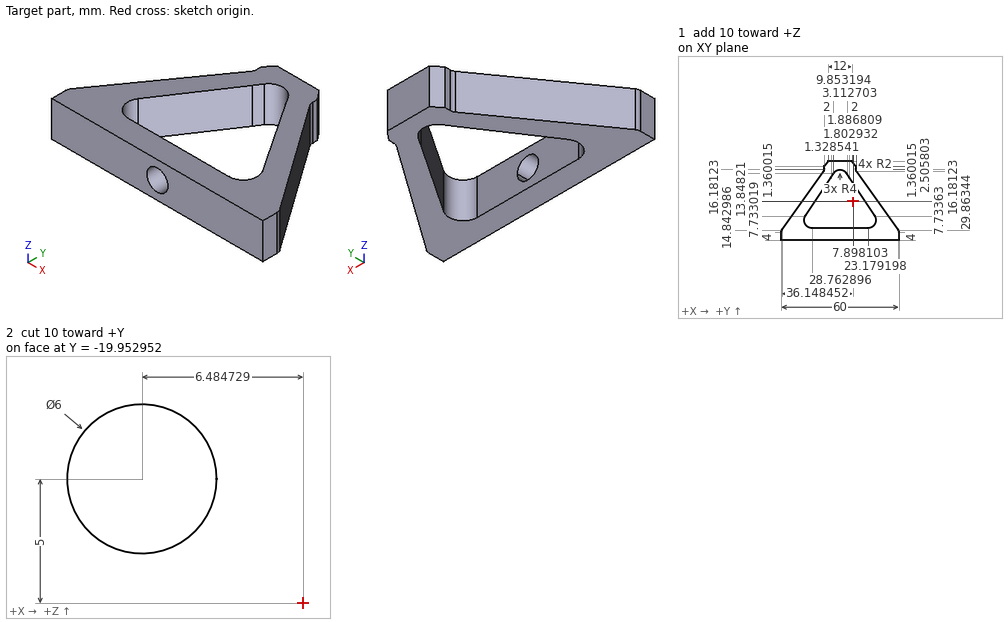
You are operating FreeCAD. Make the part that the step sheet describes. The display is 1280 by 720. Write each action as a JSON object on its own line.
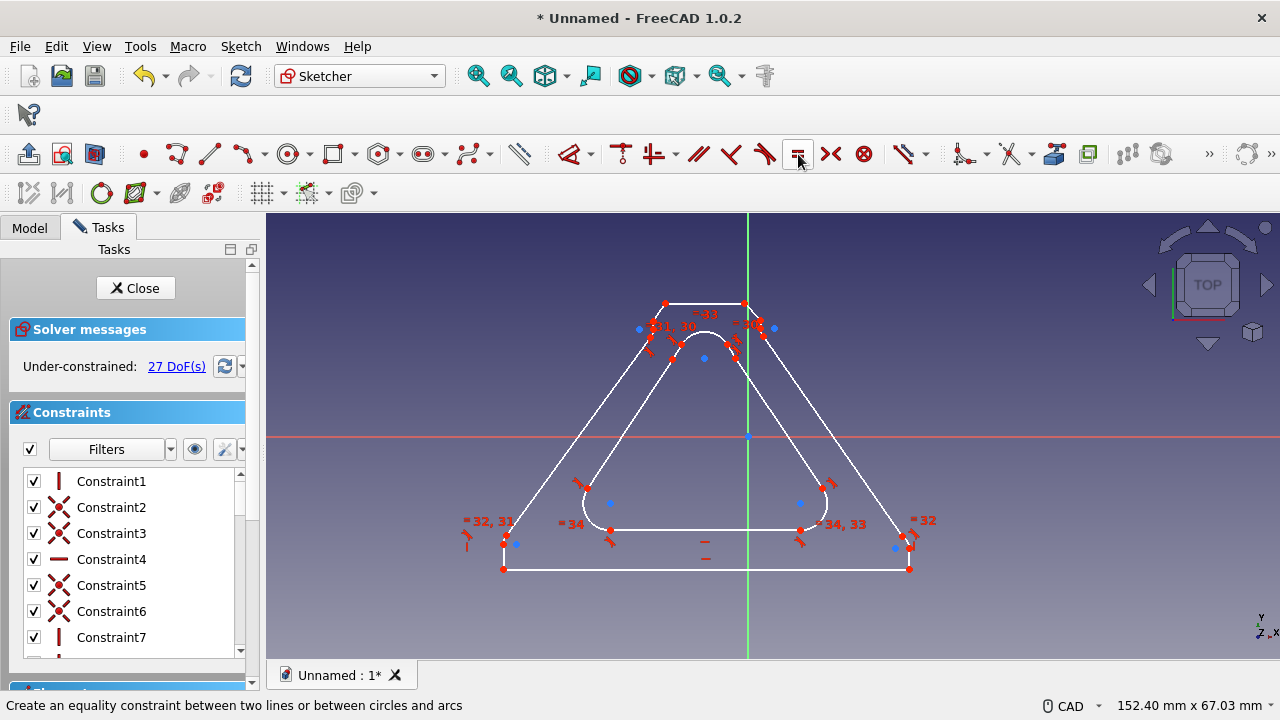
{"action": "scroll", "coordinate": [761, 333], "scroll_direction": "up", "scroll_amount": 7}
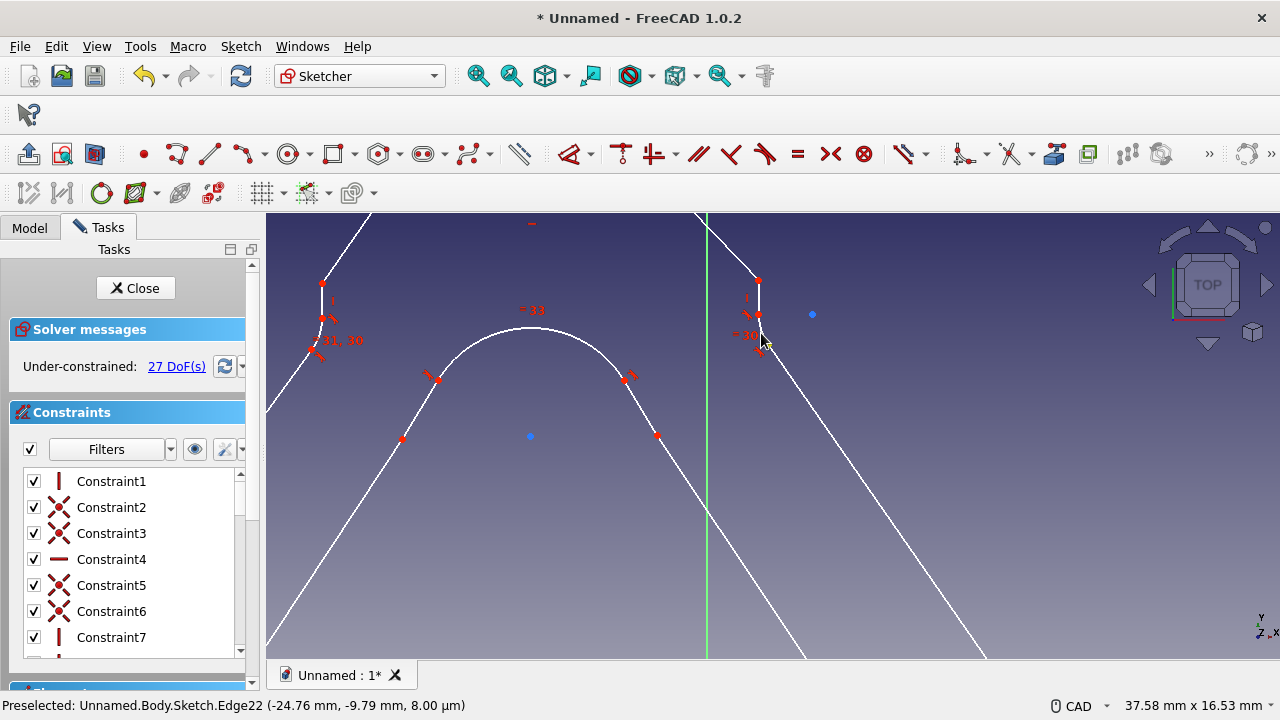
{"action": "left_click", "coordinate": [761, 330]}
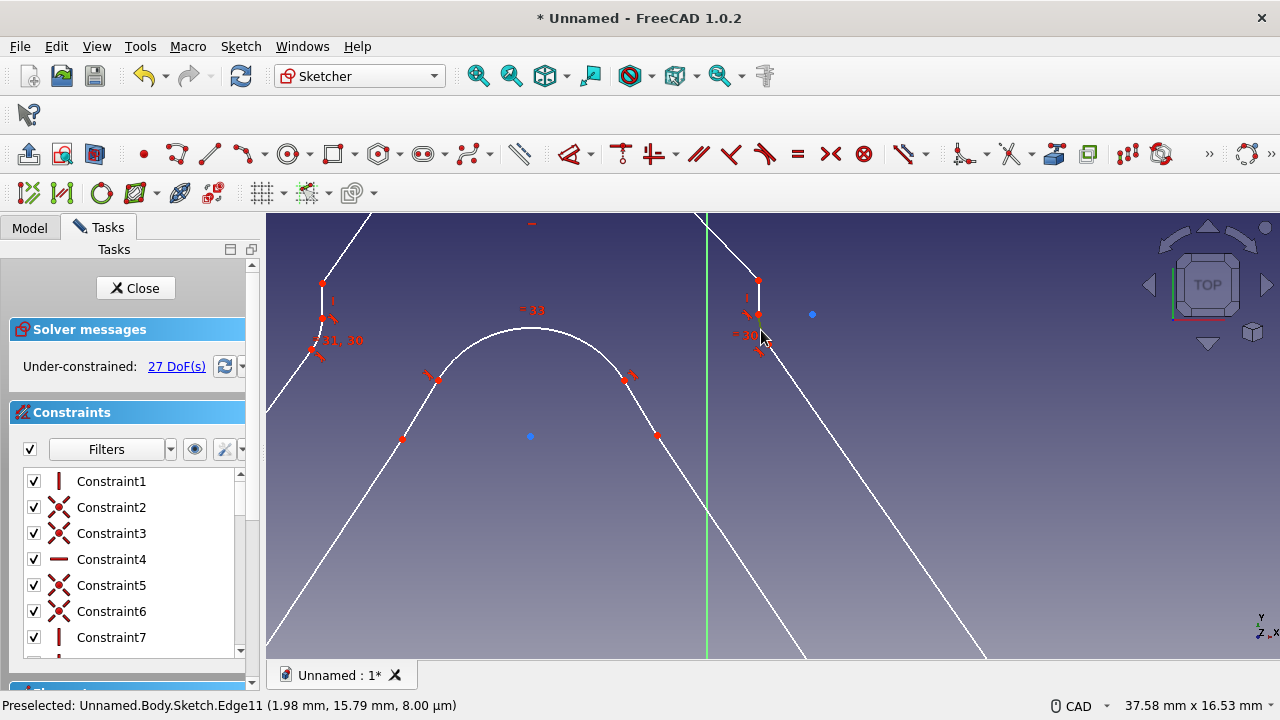
{"action": "key", "text": "k r"}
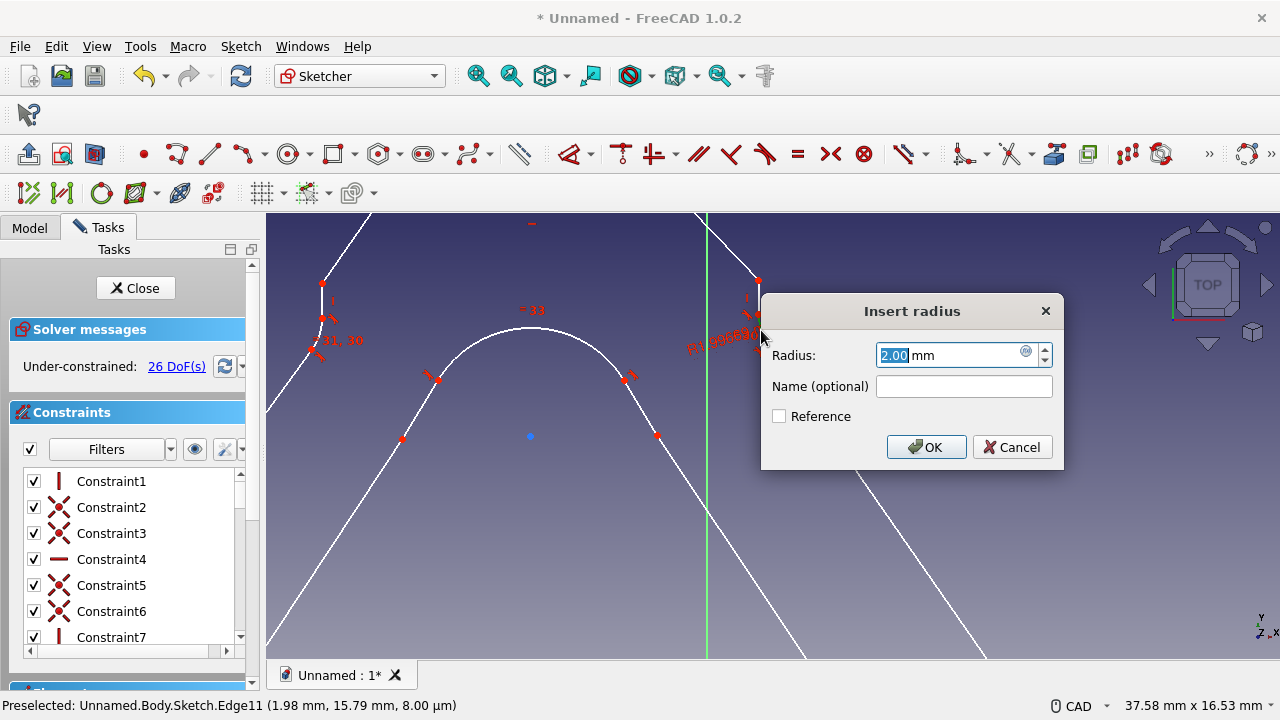
{"action": "type", "text": "2"}
{"action": "key", "text": "Return"}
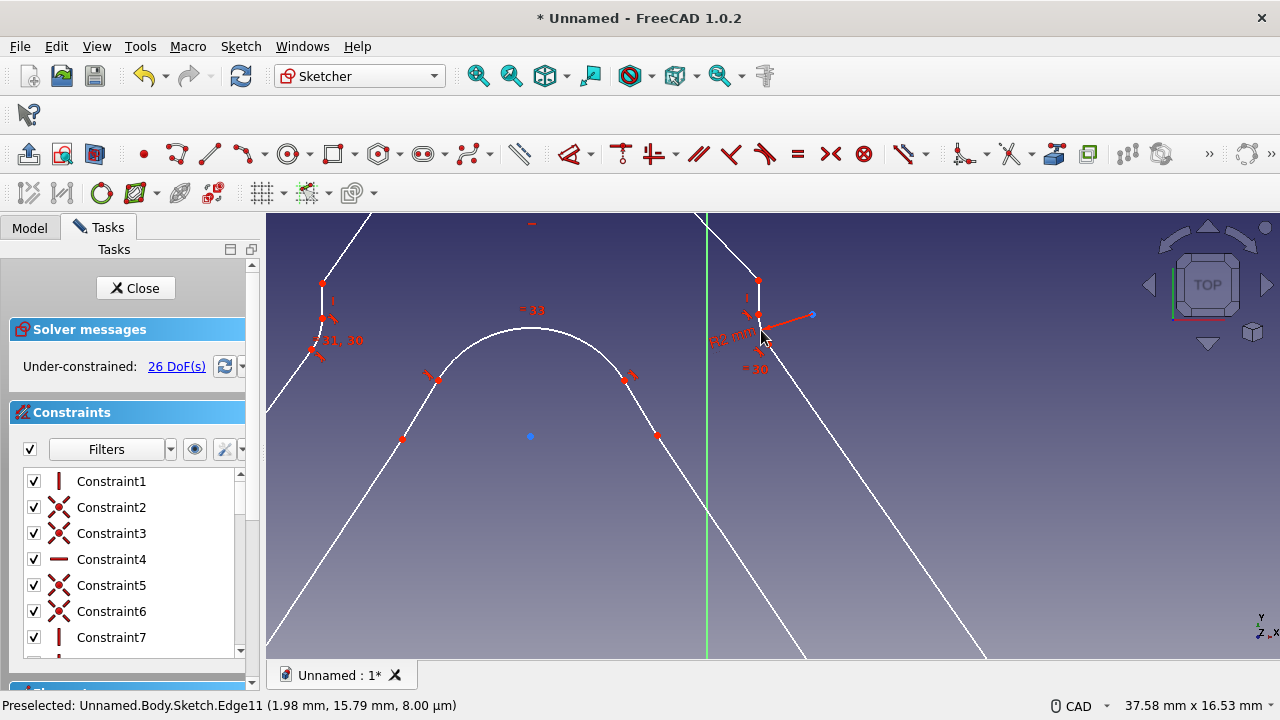
{"action": "left_click", "coordinate": [575, 337]}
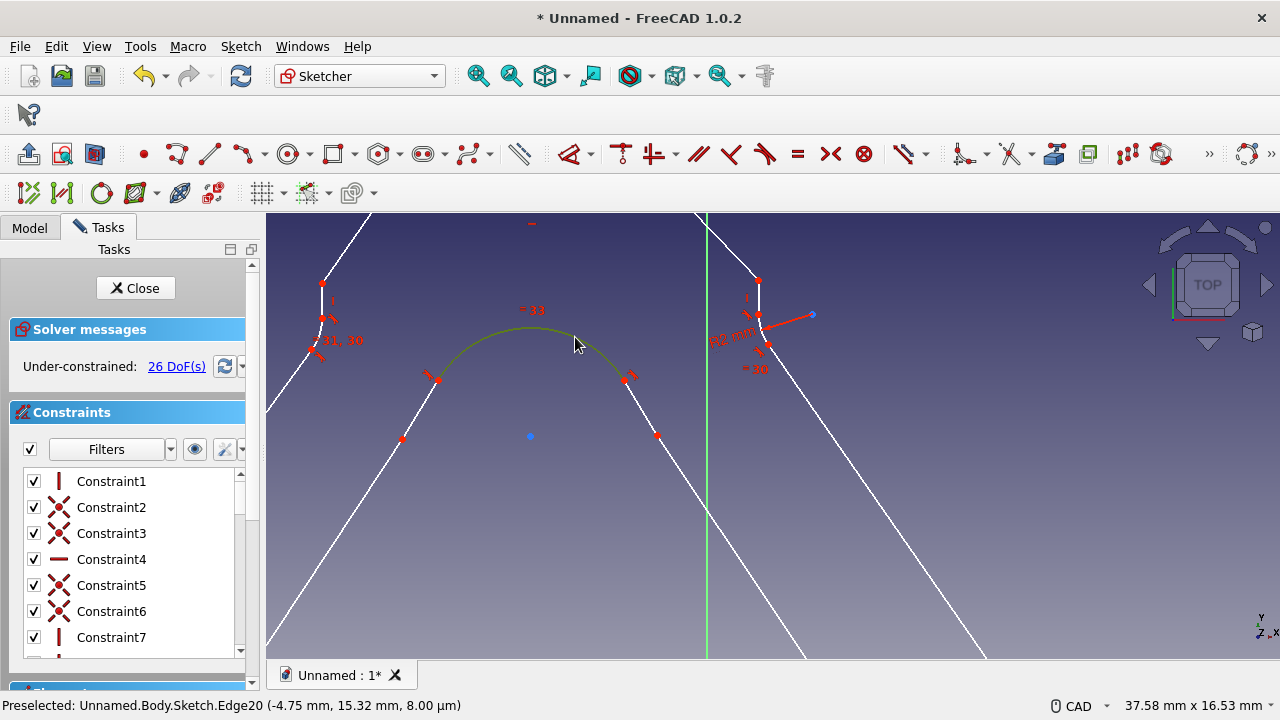
{"action": "key", "text": "k r"}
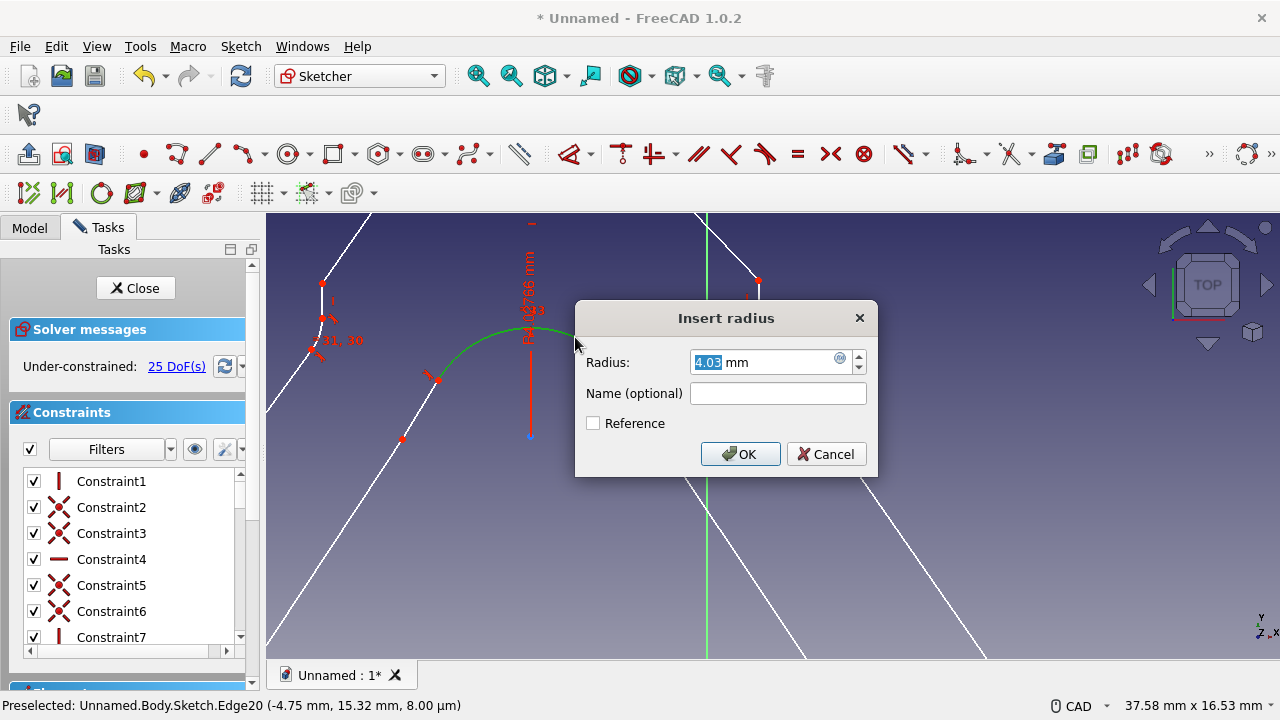
{"action": "type", "text": "4"}
{"action": "key", "text": "Return"}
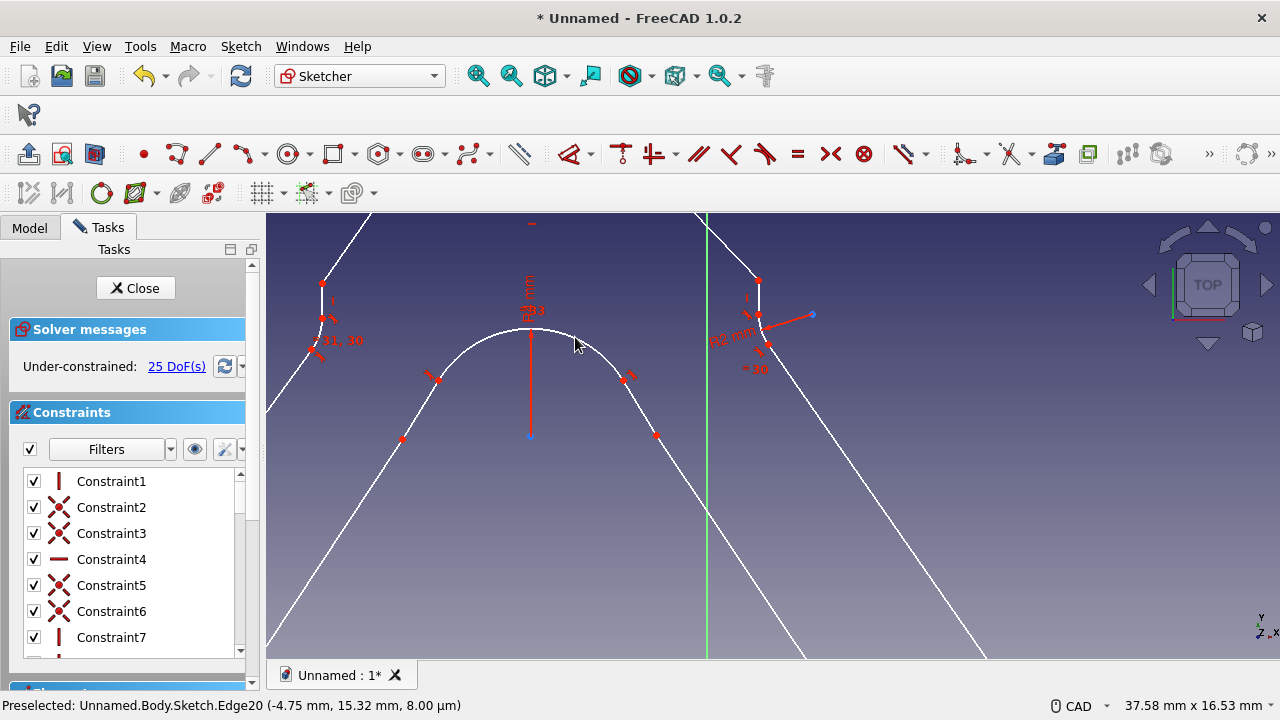
{"action": "scroll", "coordinate": [761, 333], "scroll_direction": "down", "scroll_amount": 7}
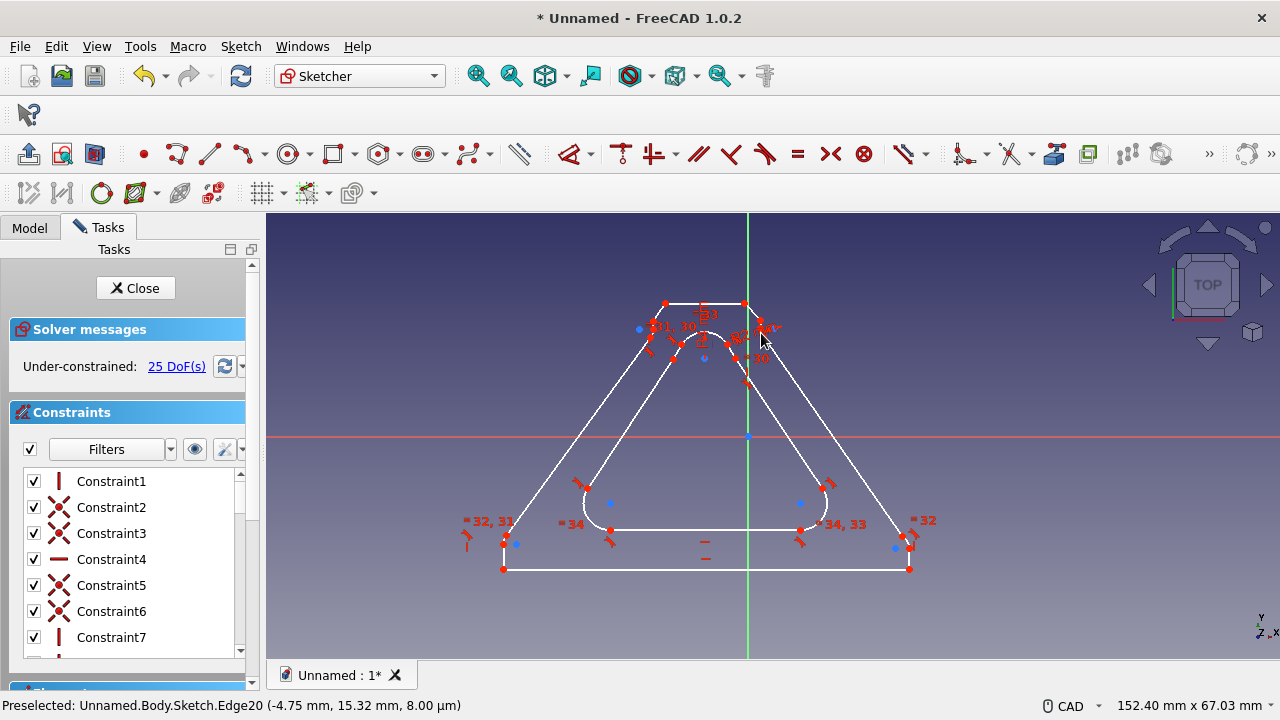
{"action": "scroll", "coordinate": [504, 552], "scroll_direction": "up", "scroll_amount": 3}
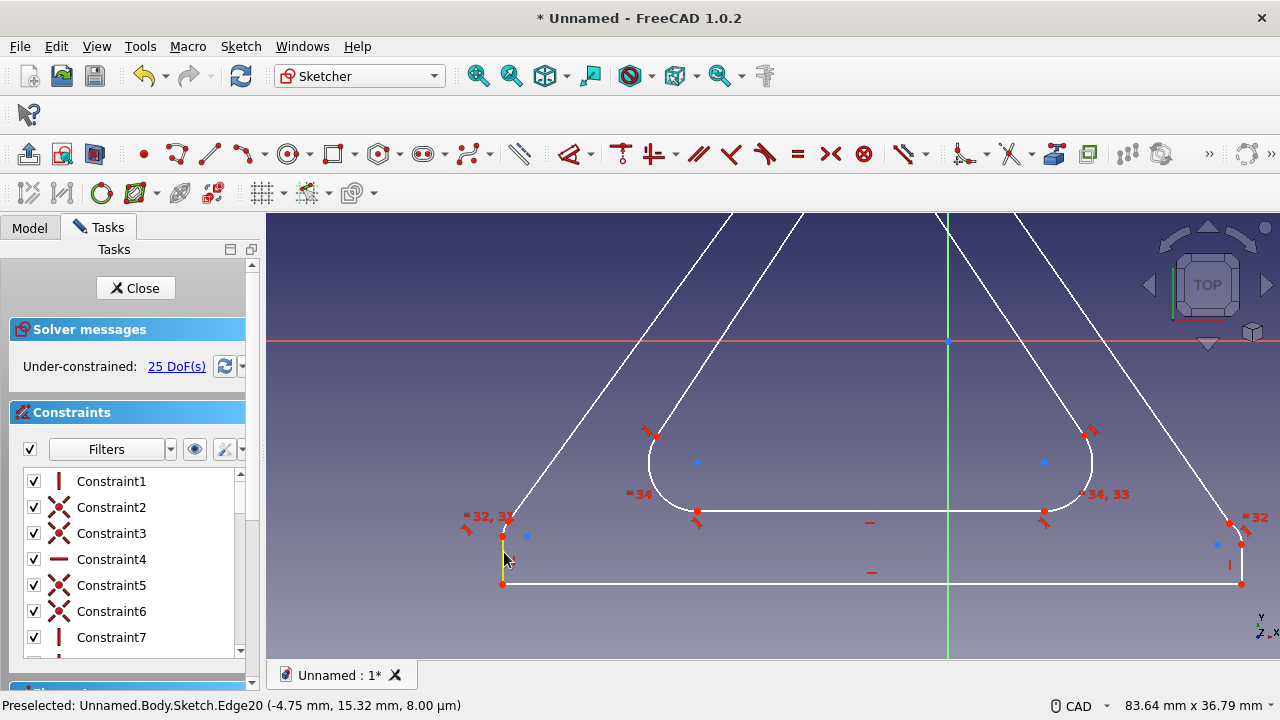
{"action": "left_click", "coordinate": [503, 551]}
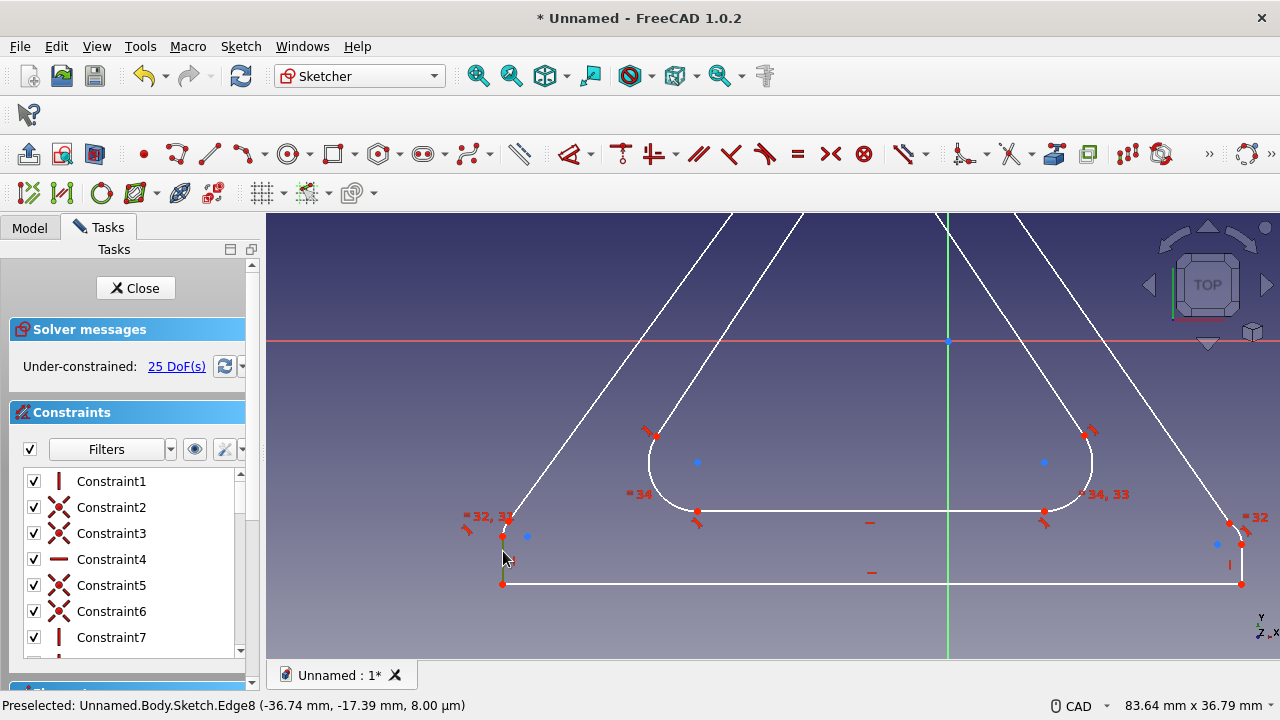
{"action": "left_click", "coordinate": [590, 154]}